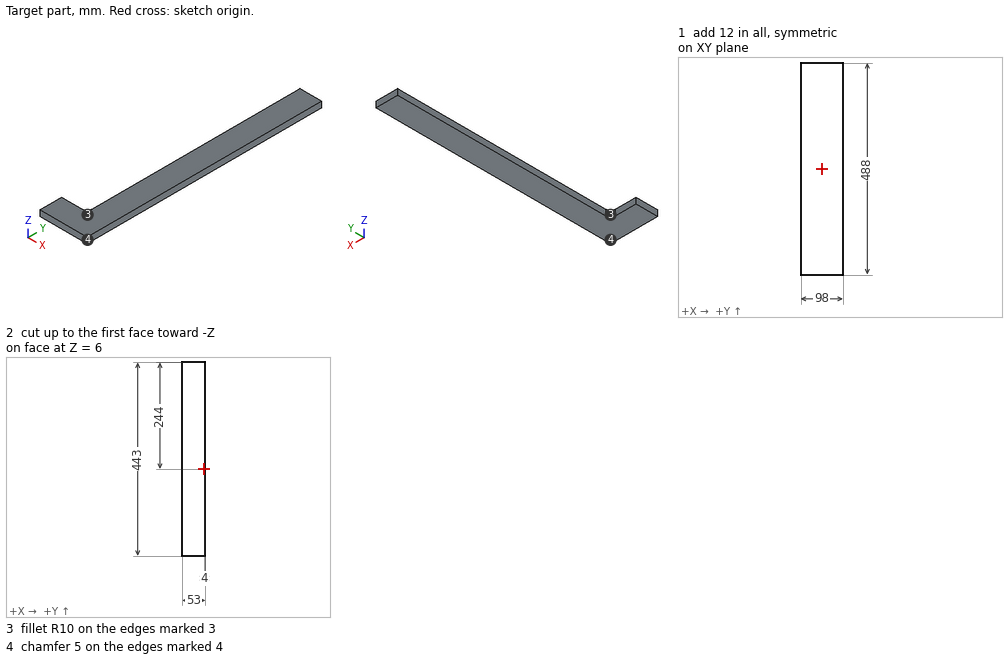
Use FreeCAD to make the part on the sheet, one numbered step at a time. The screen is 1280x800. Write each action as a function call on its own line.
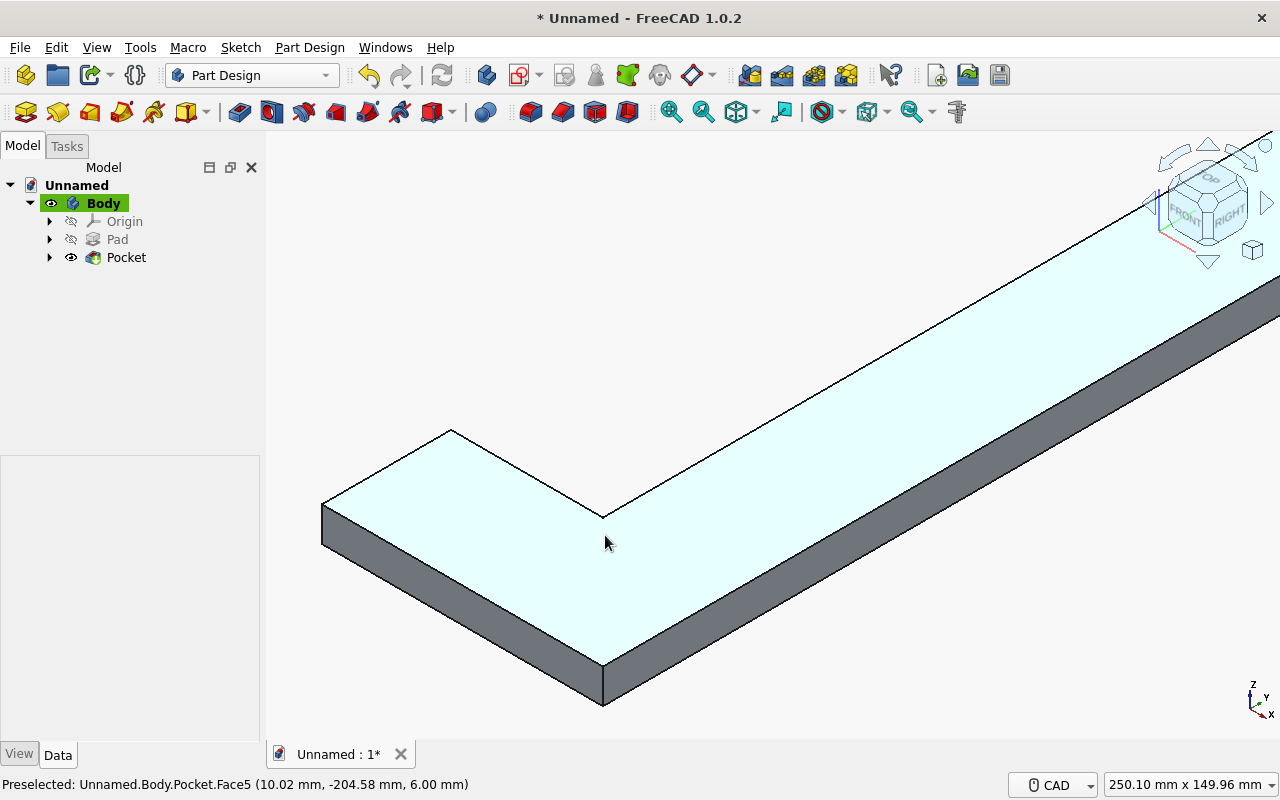
key(v)
key(f)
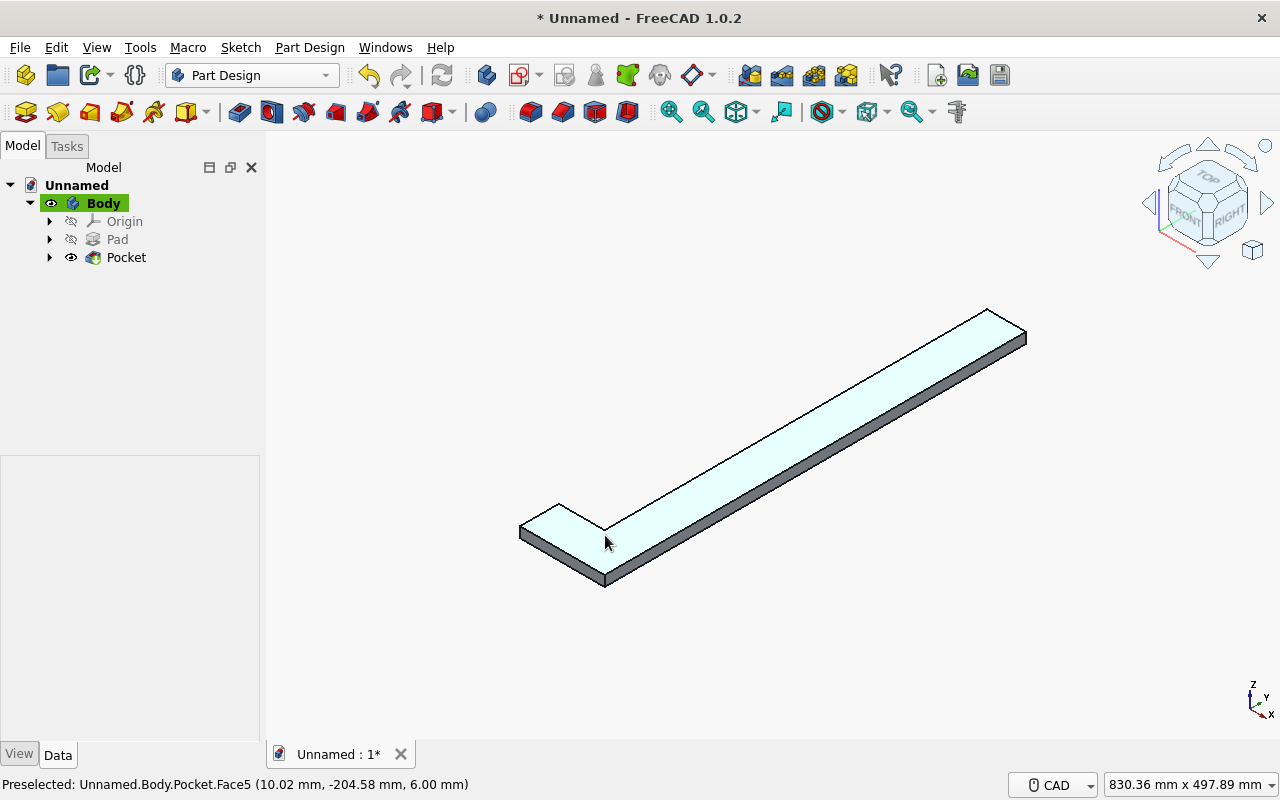
key(2)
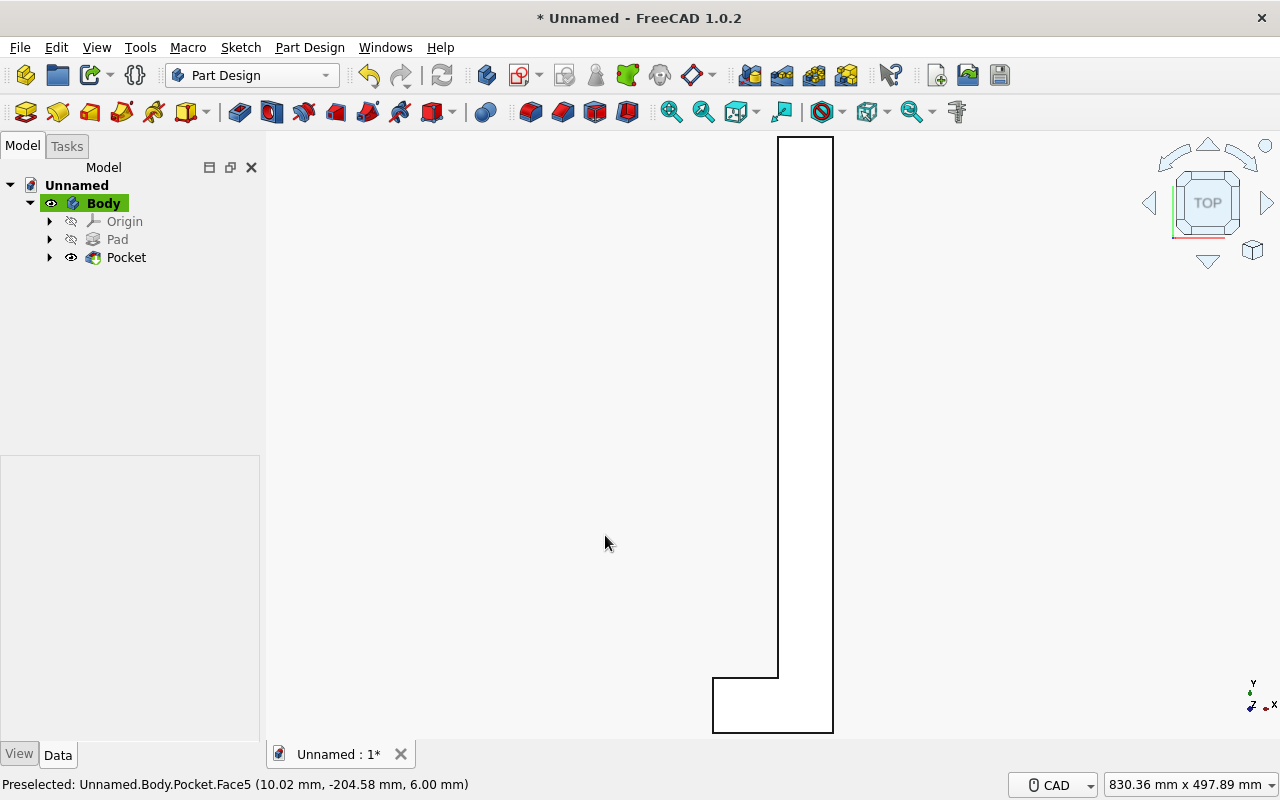
scroll(778, 677, up, 6)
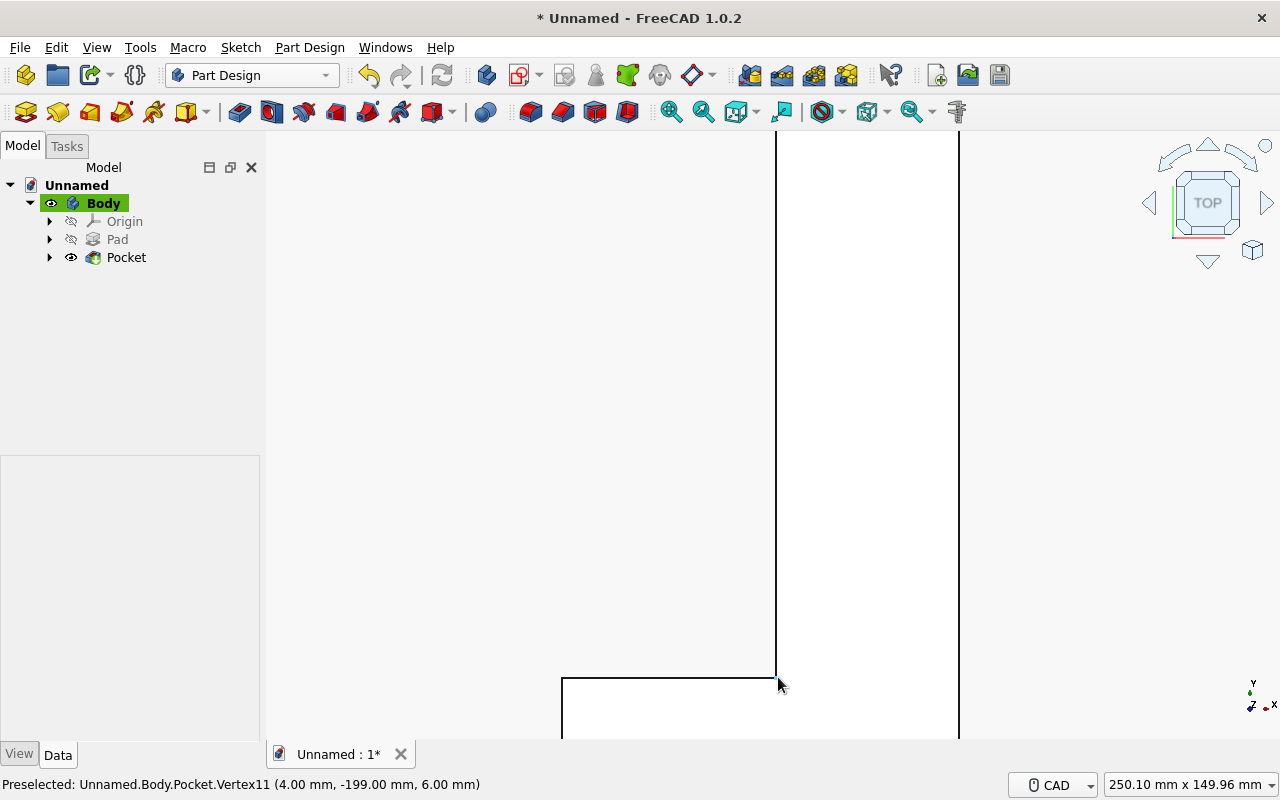
key(v)
key(f)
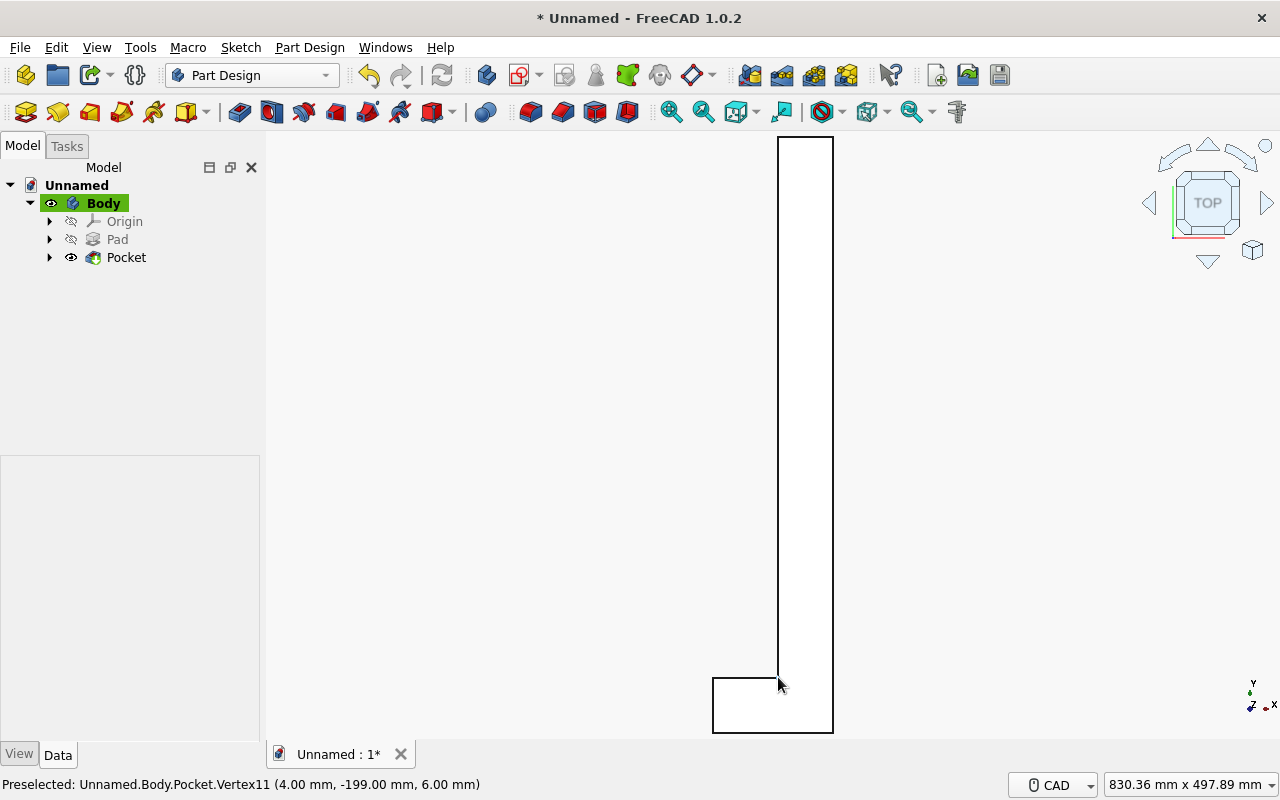
key(1)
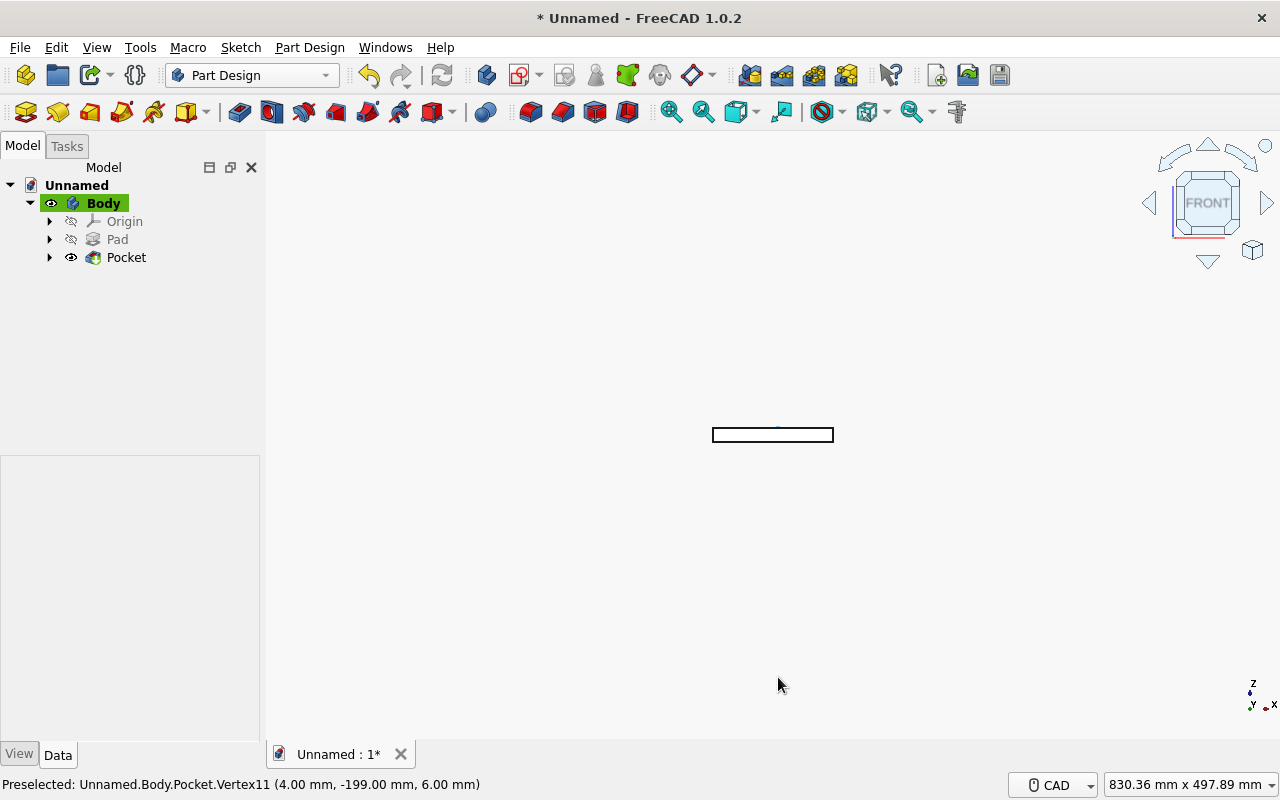
key(v)
key(f)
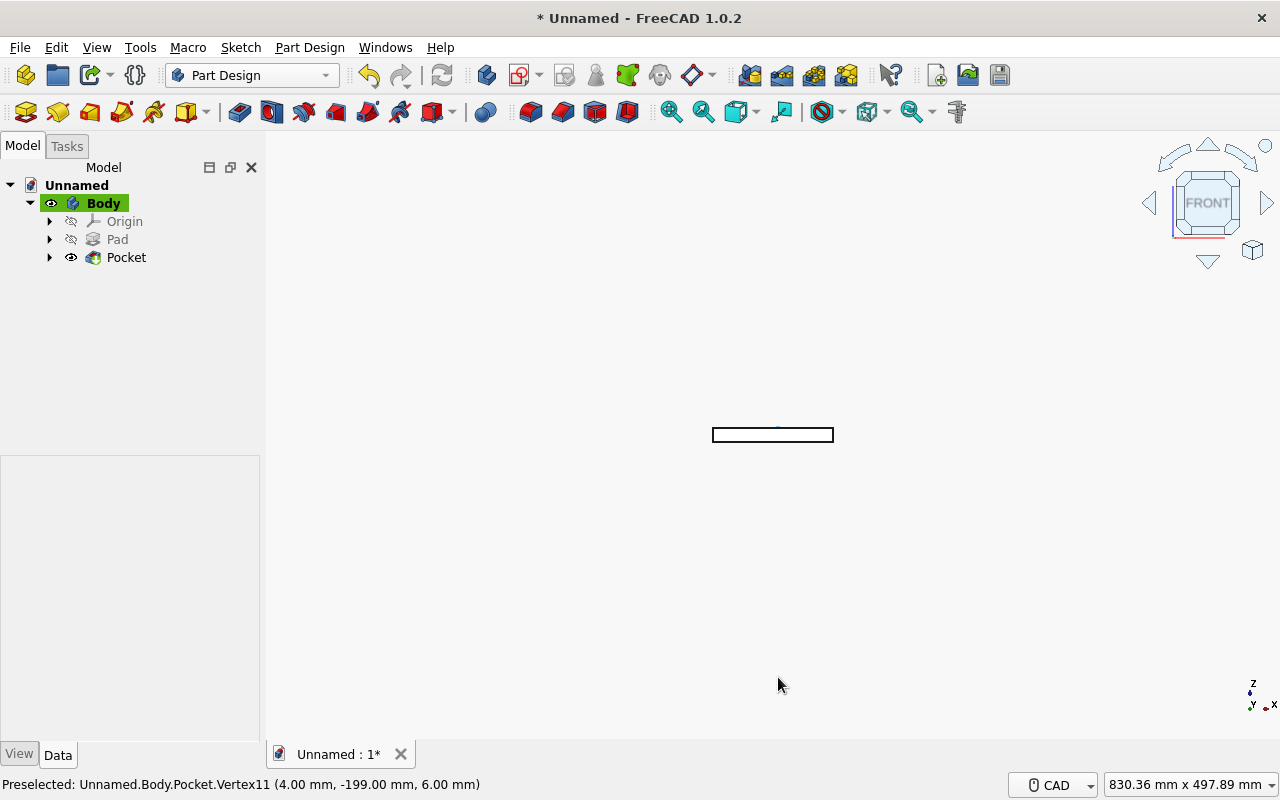
scroll(778, 434, up, 6)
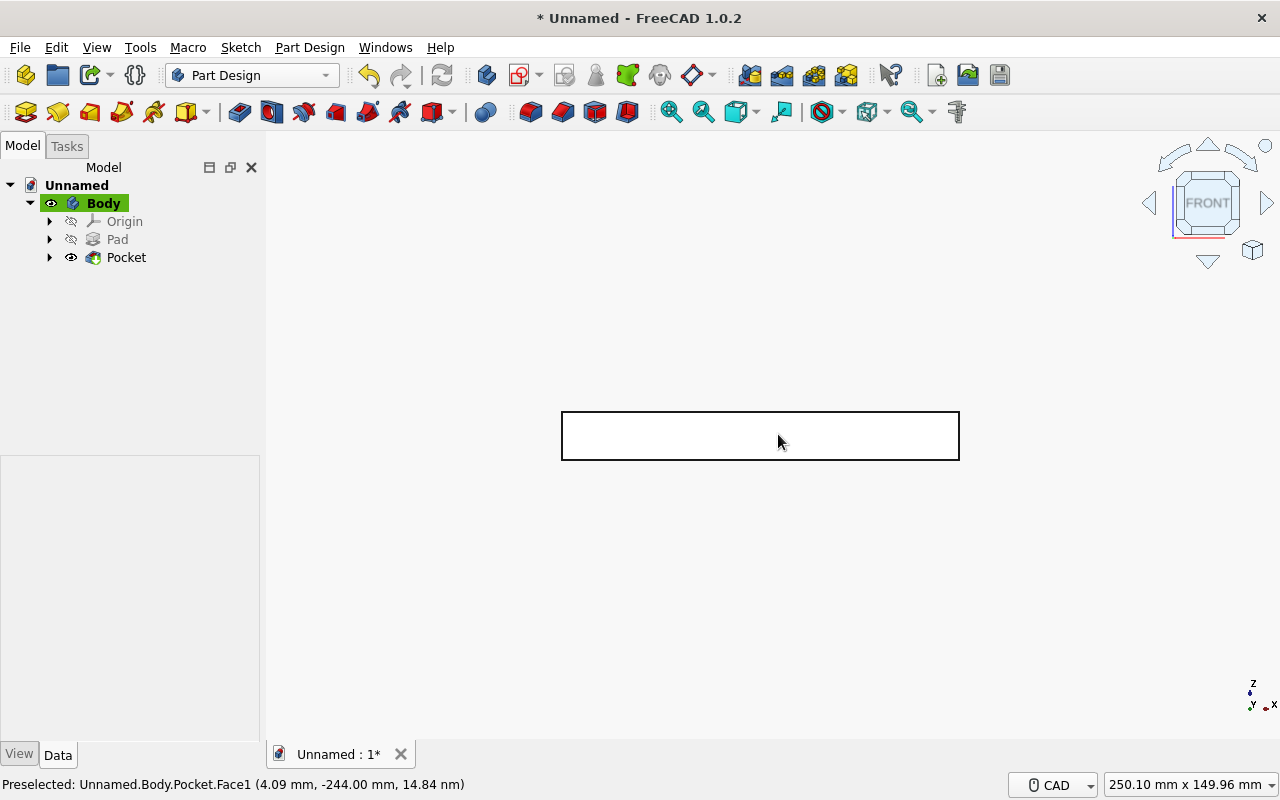
key(v)
key(f)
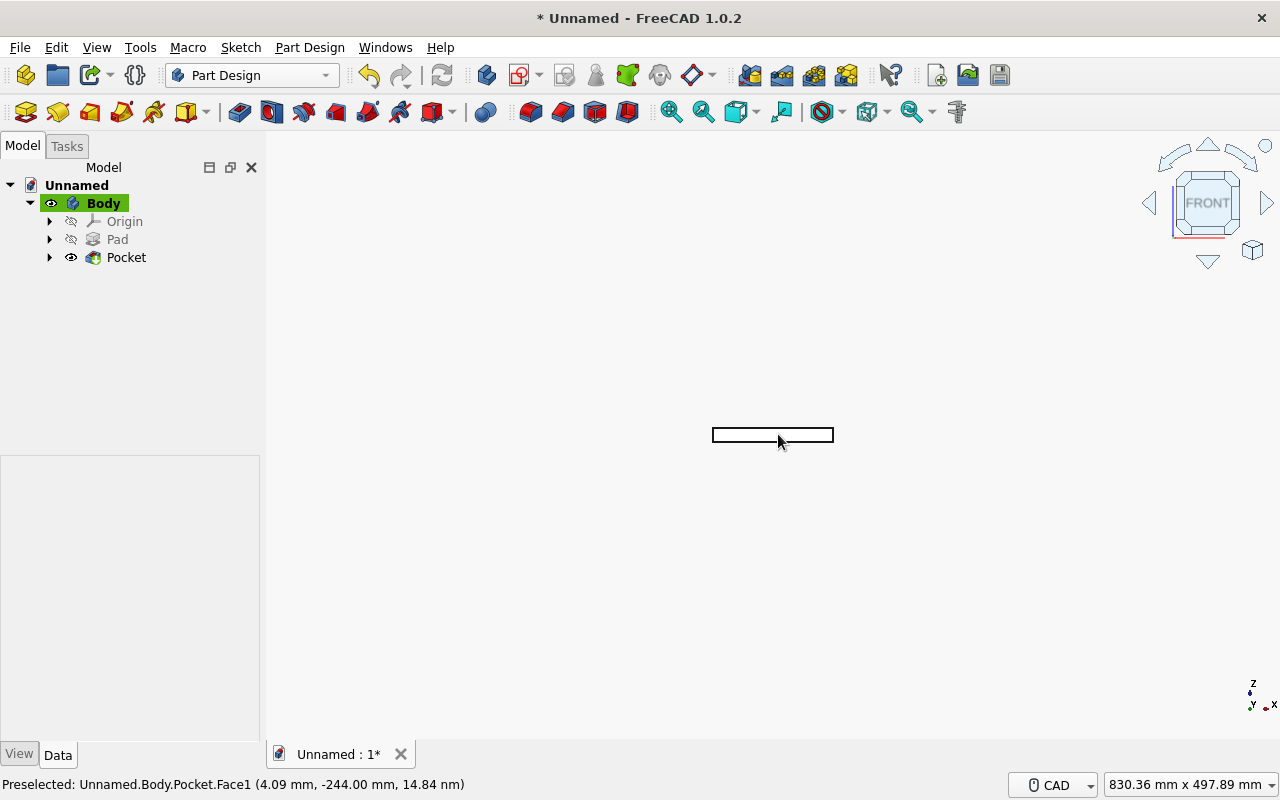
key(3)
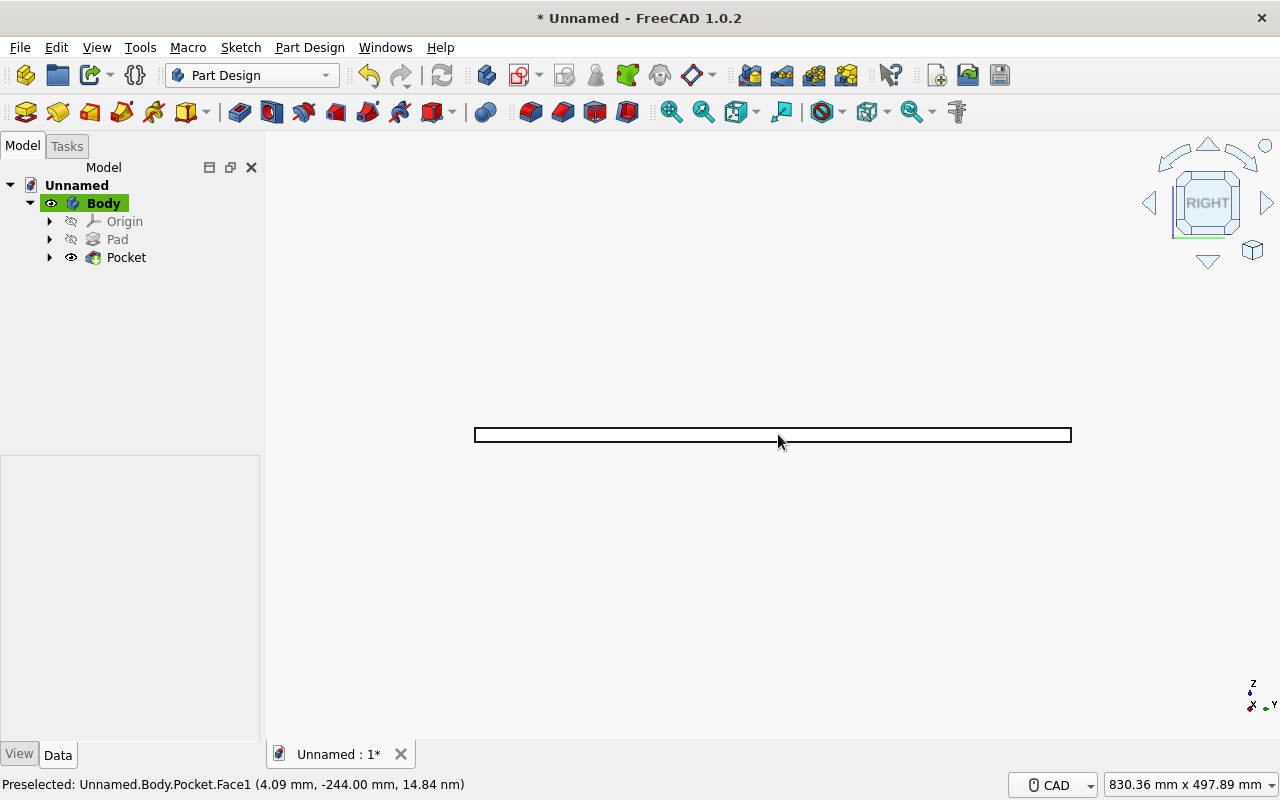
scroll(530, 434, up, 6)